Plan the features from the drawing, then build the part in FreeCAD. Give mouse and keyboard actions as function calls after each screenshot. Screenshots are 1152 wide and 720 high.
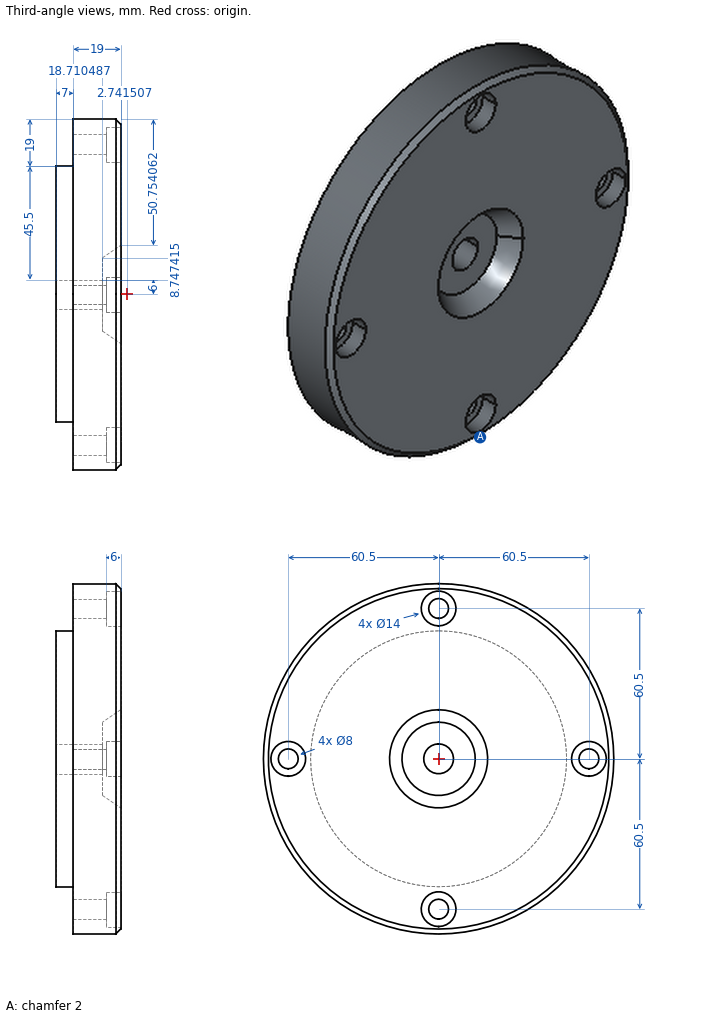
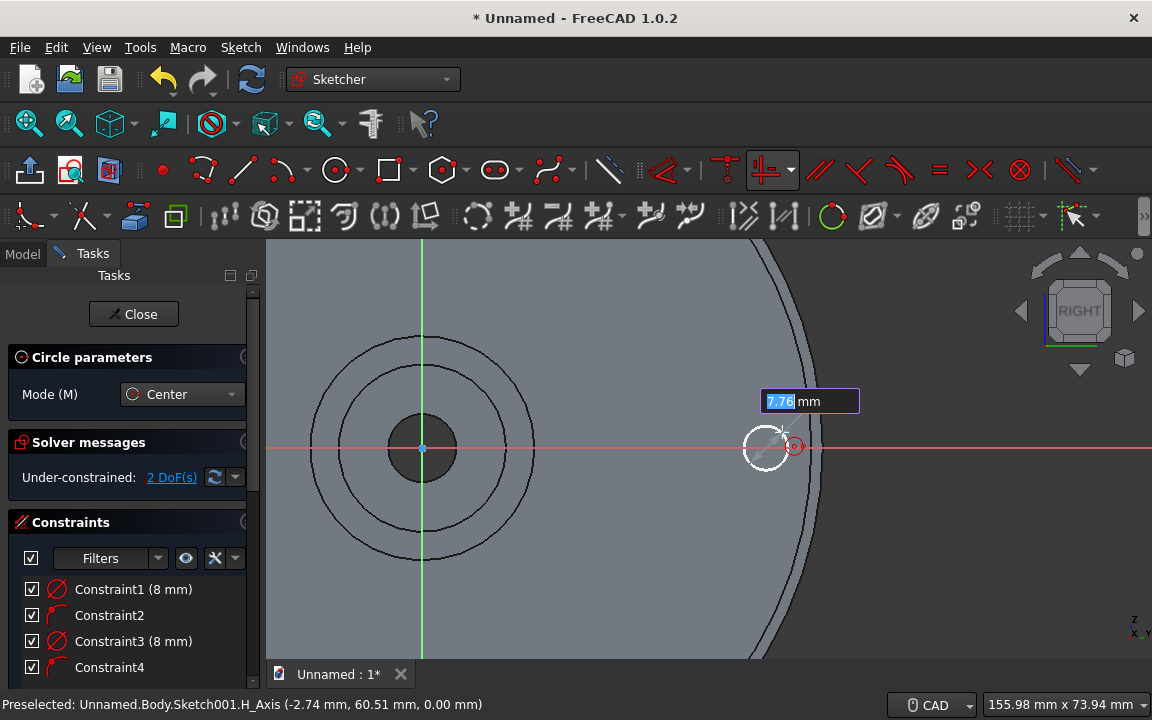
text(8)
key(Return)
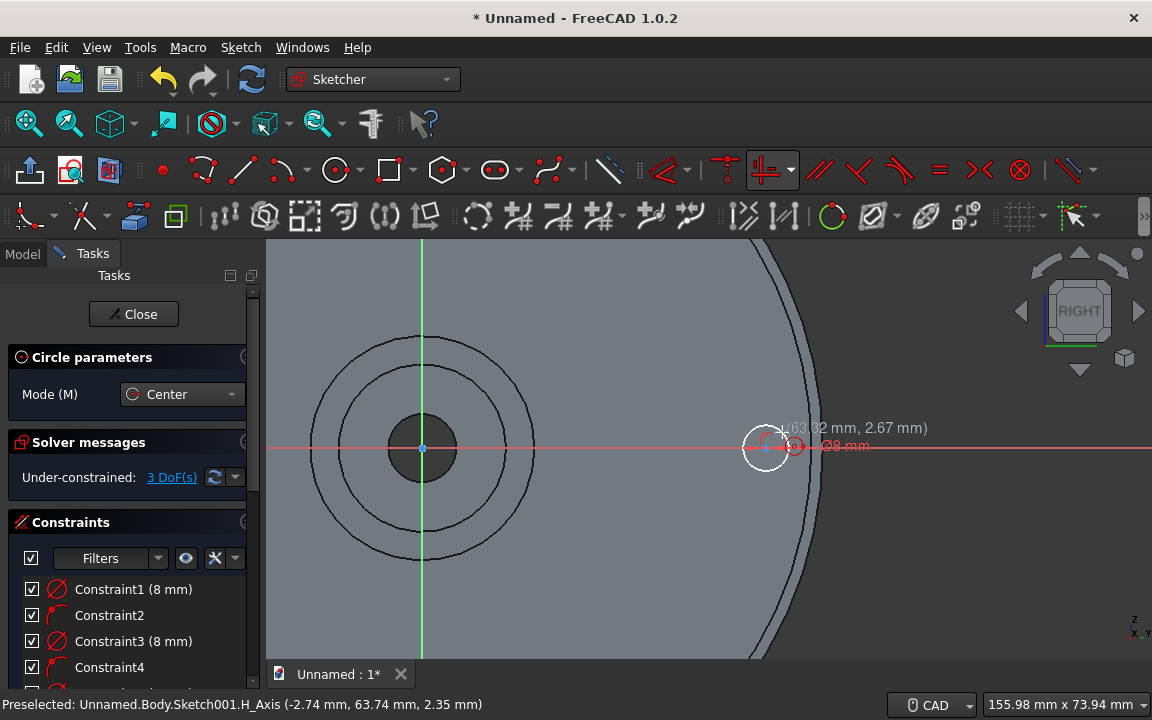
scroll(767, 450, down, 5)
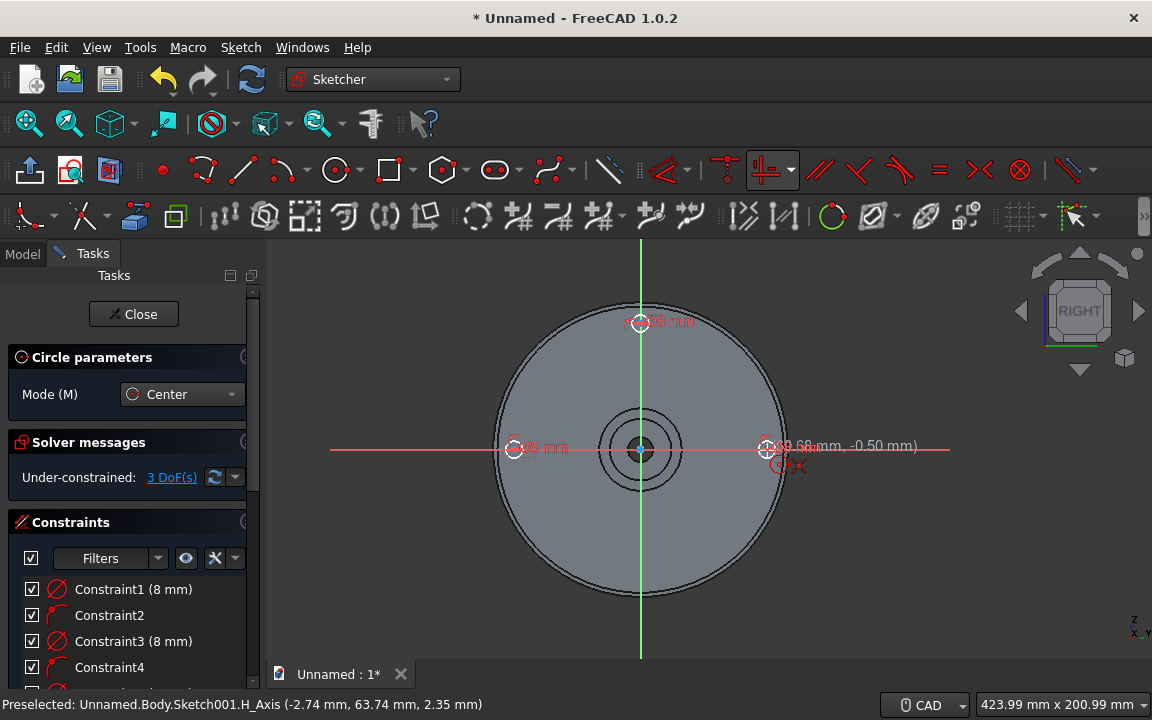
scroll(641, 576, up, 5)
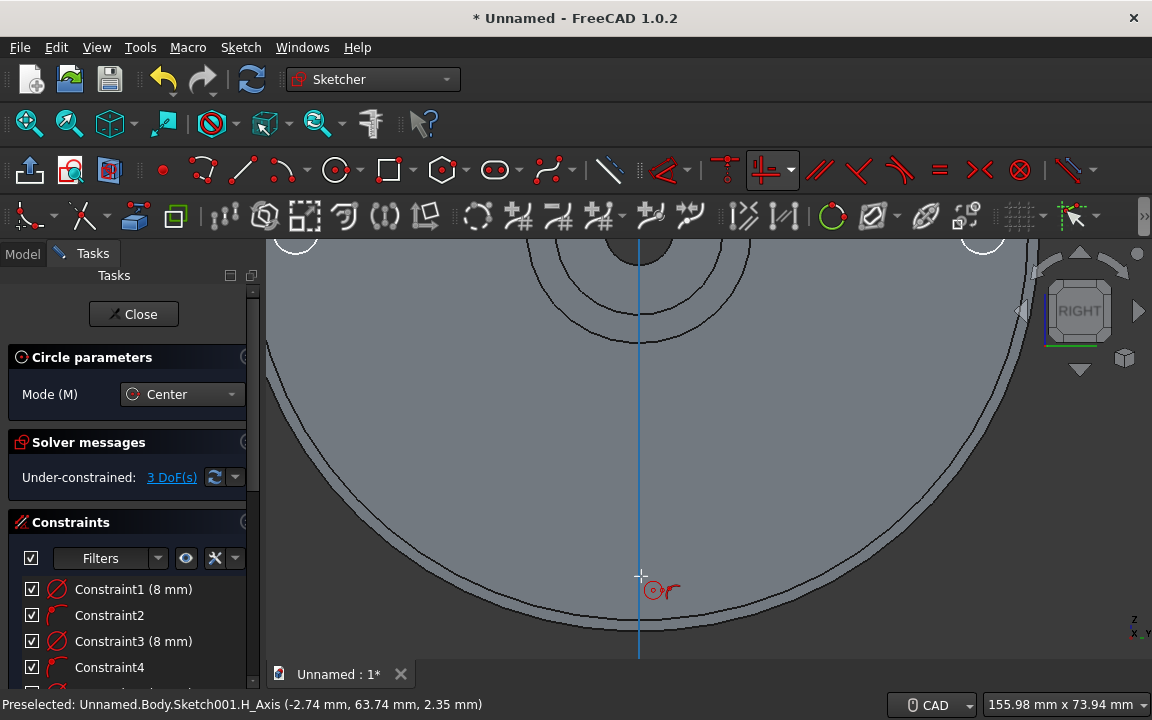
click(639, 575)
move(655, 559)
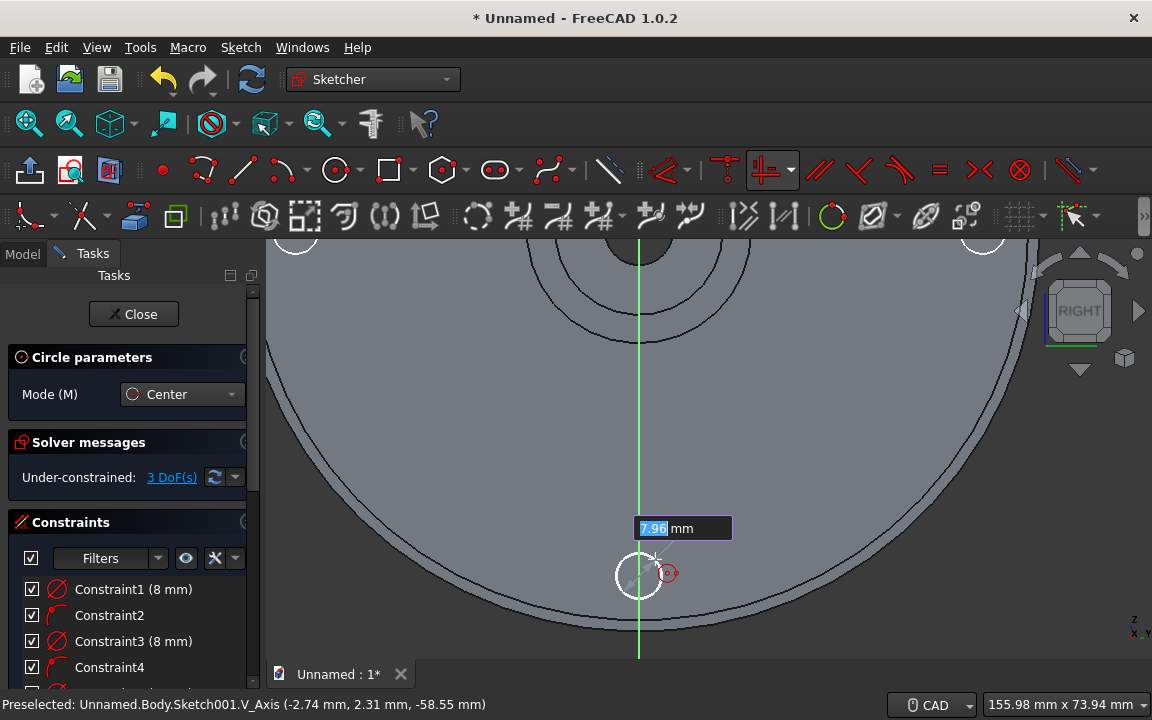
text(8)
key(Return)
key(Escape)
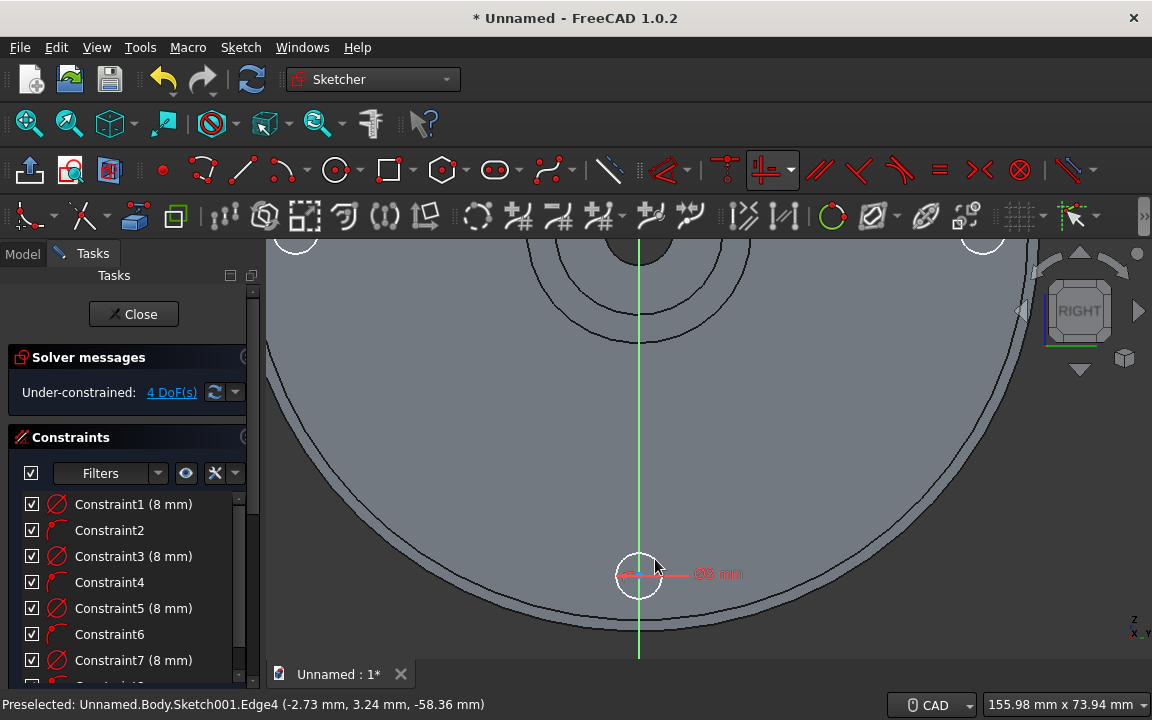
key(d)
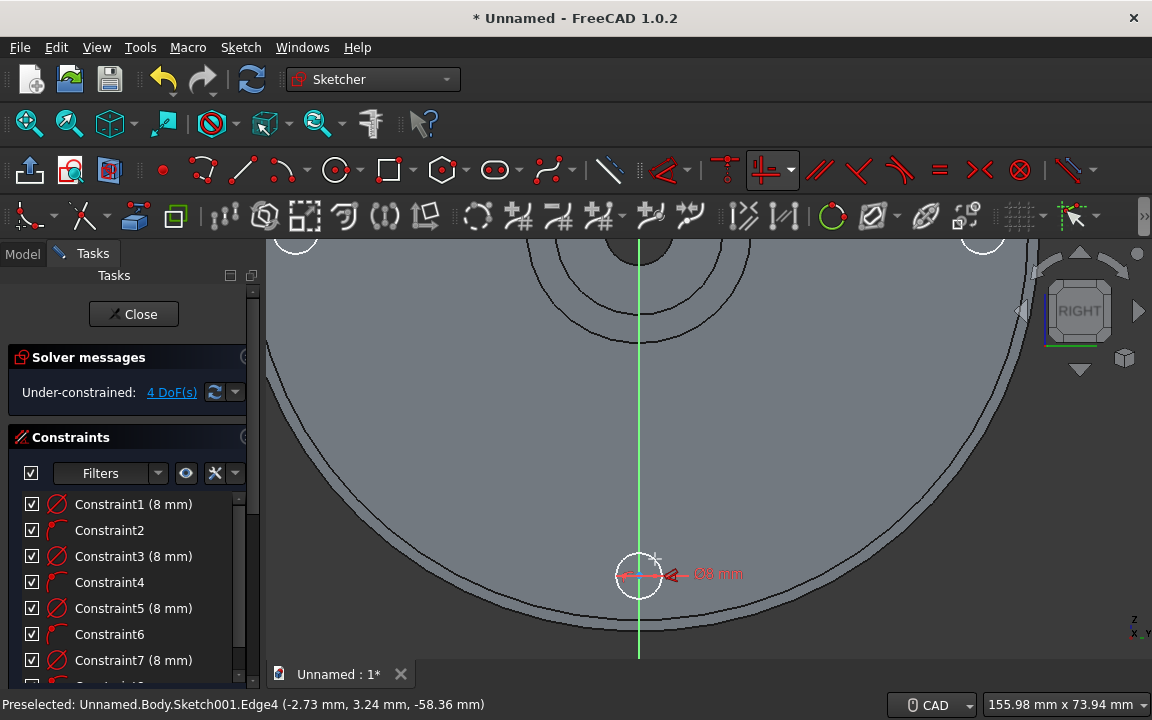
scroll(641, 576, down, 5)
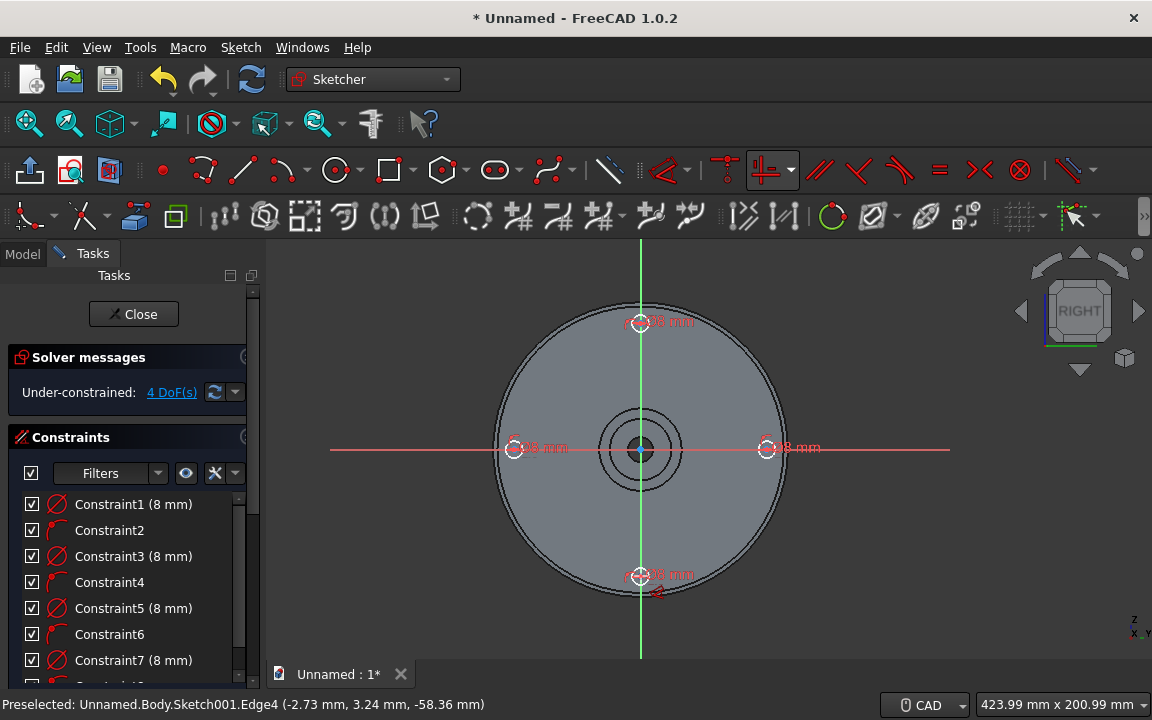
click(514, 450)
click(577, 484)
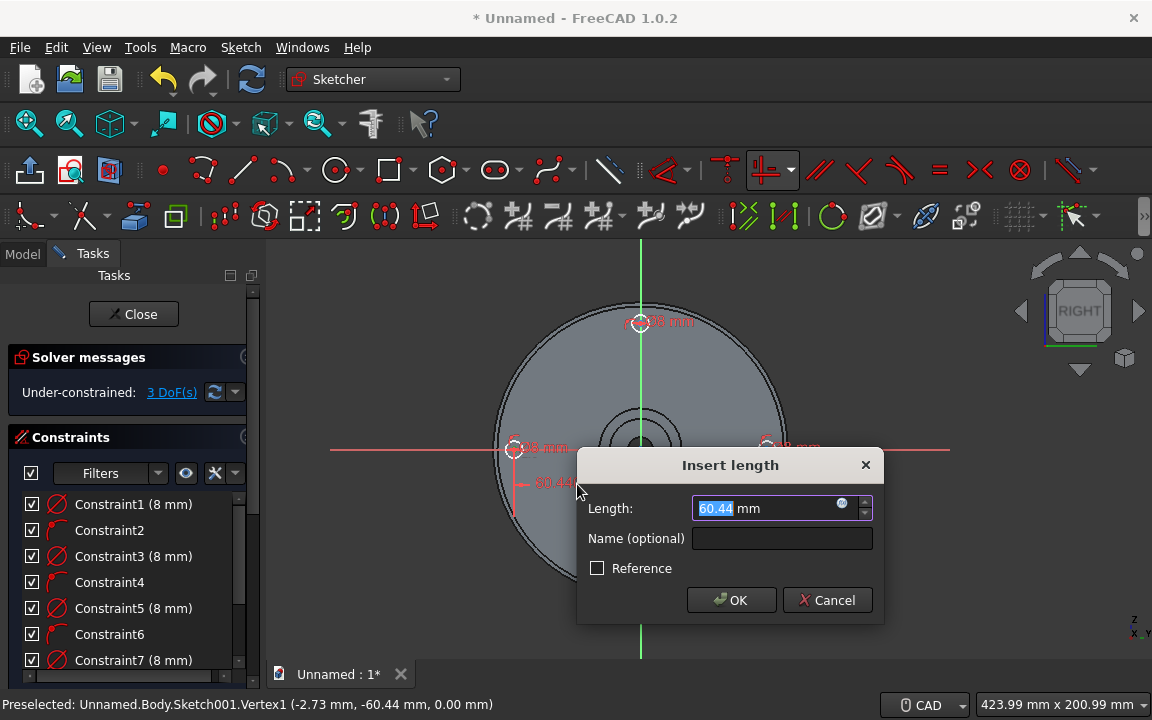
text(60.5)
key(Return)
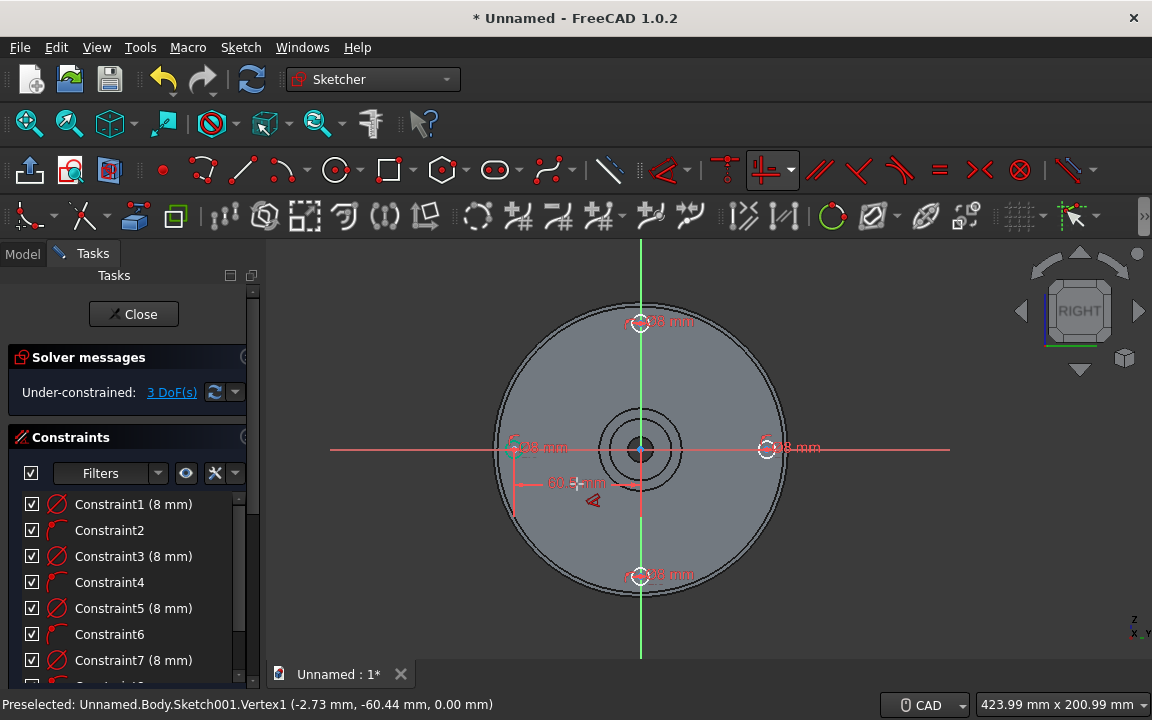
click(641, 323)
click(675, 387)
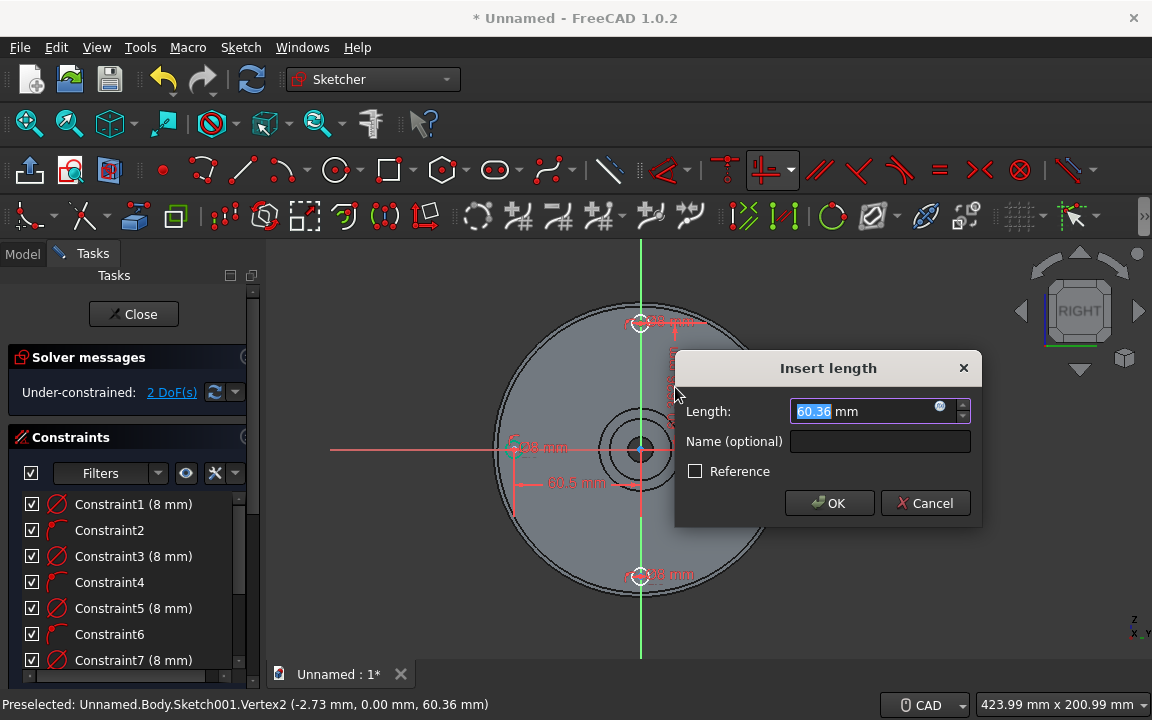
text(60.5)
key(Return)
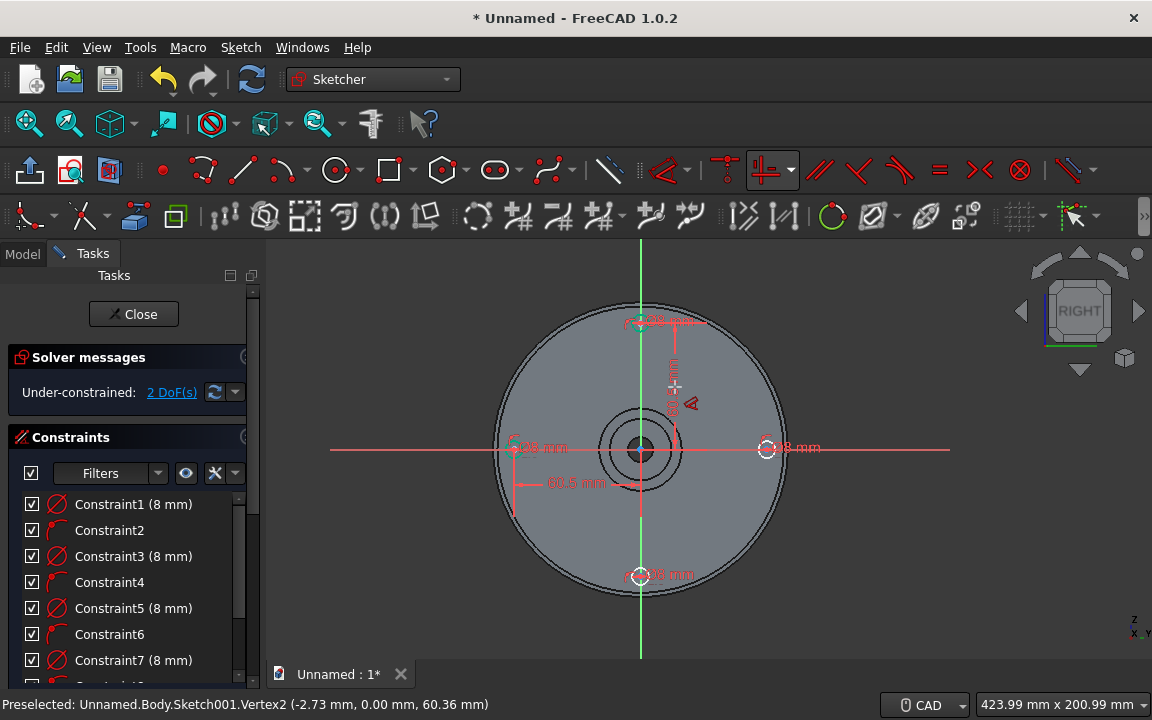
click(767, 450)
click(704, 484)